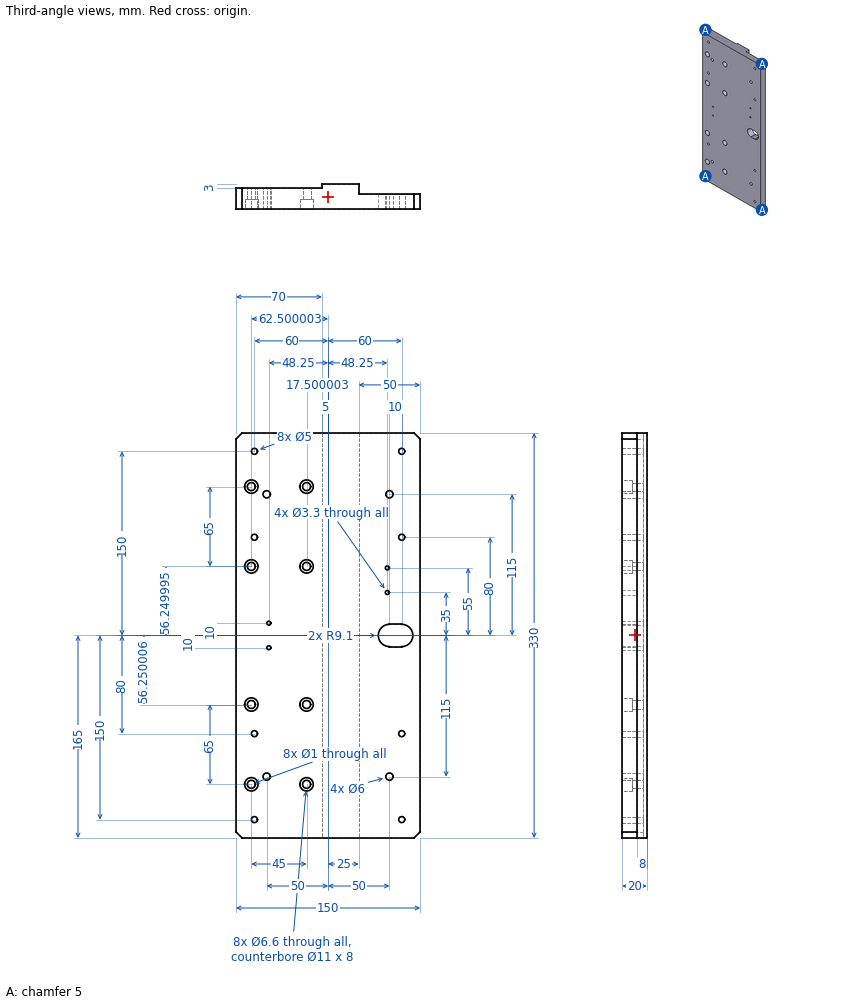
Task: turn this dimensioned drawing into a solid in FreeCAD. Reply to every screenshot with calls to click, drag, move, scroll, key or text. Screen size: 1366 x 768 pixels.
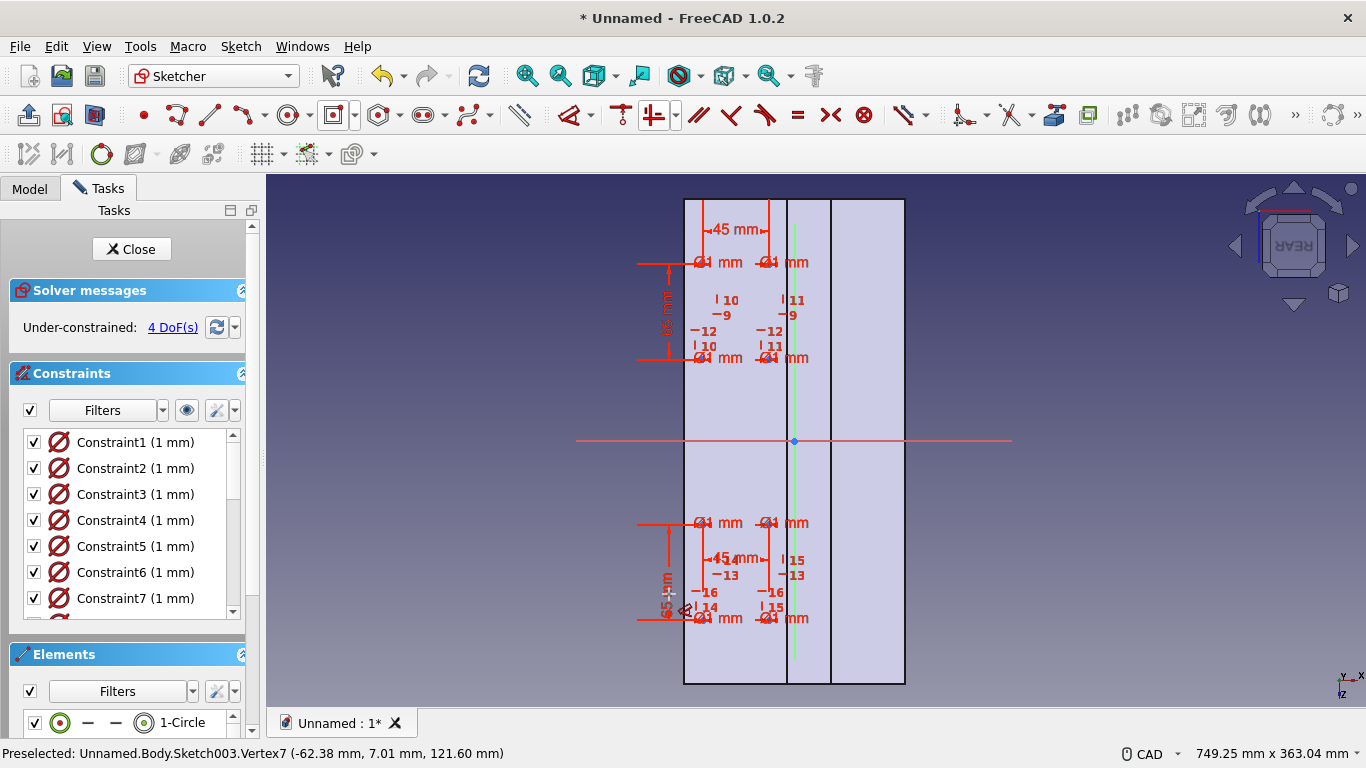
click(703, 264)
click(749, 475)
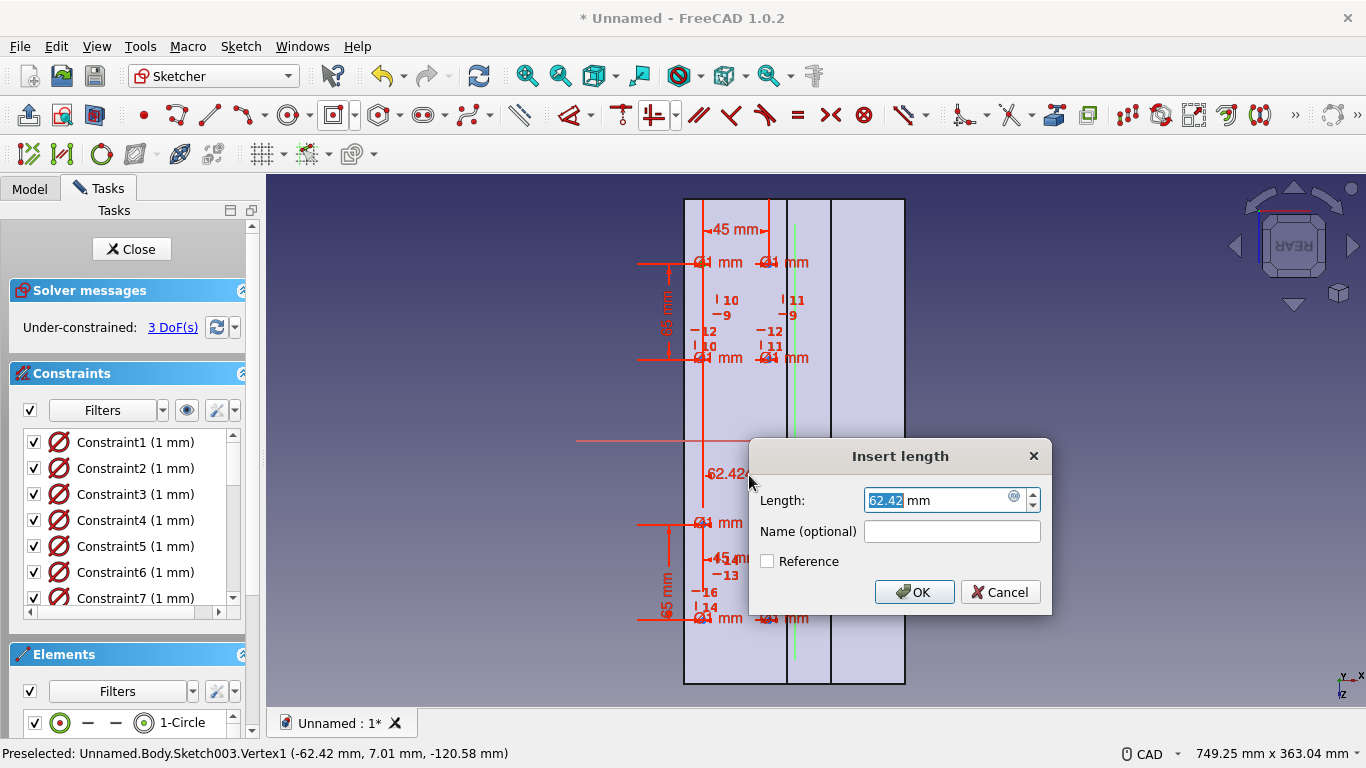
text(62.500006)
key(Return)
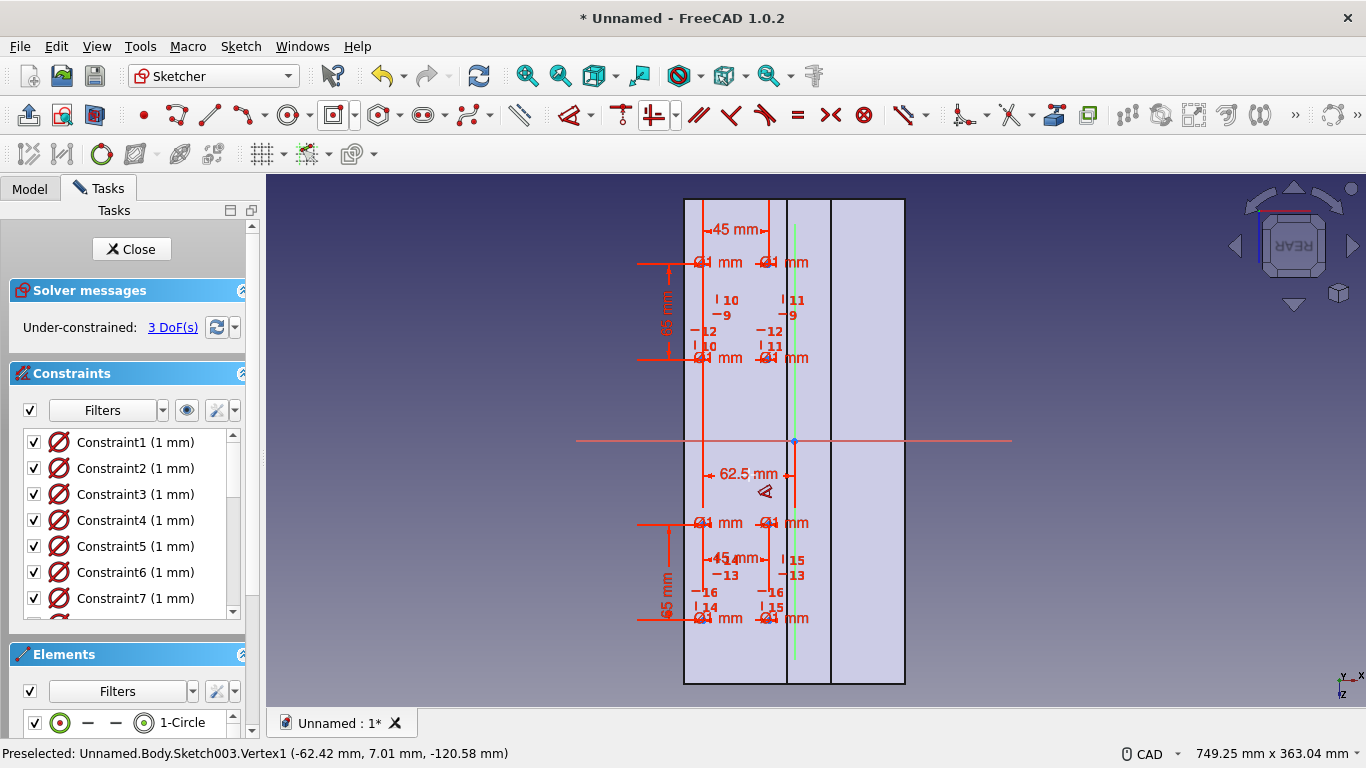
click(703, 360)
click(829, 401)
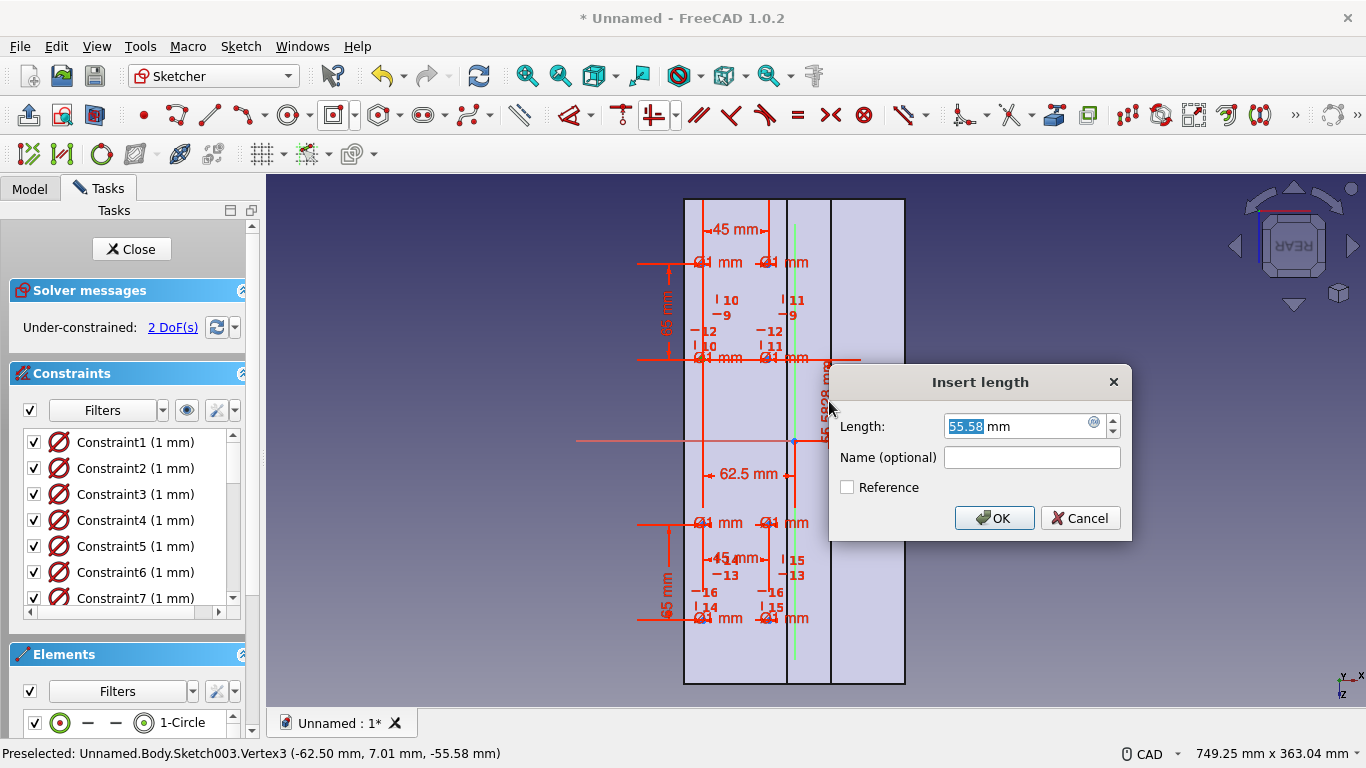
text(56.250006)
key(Return)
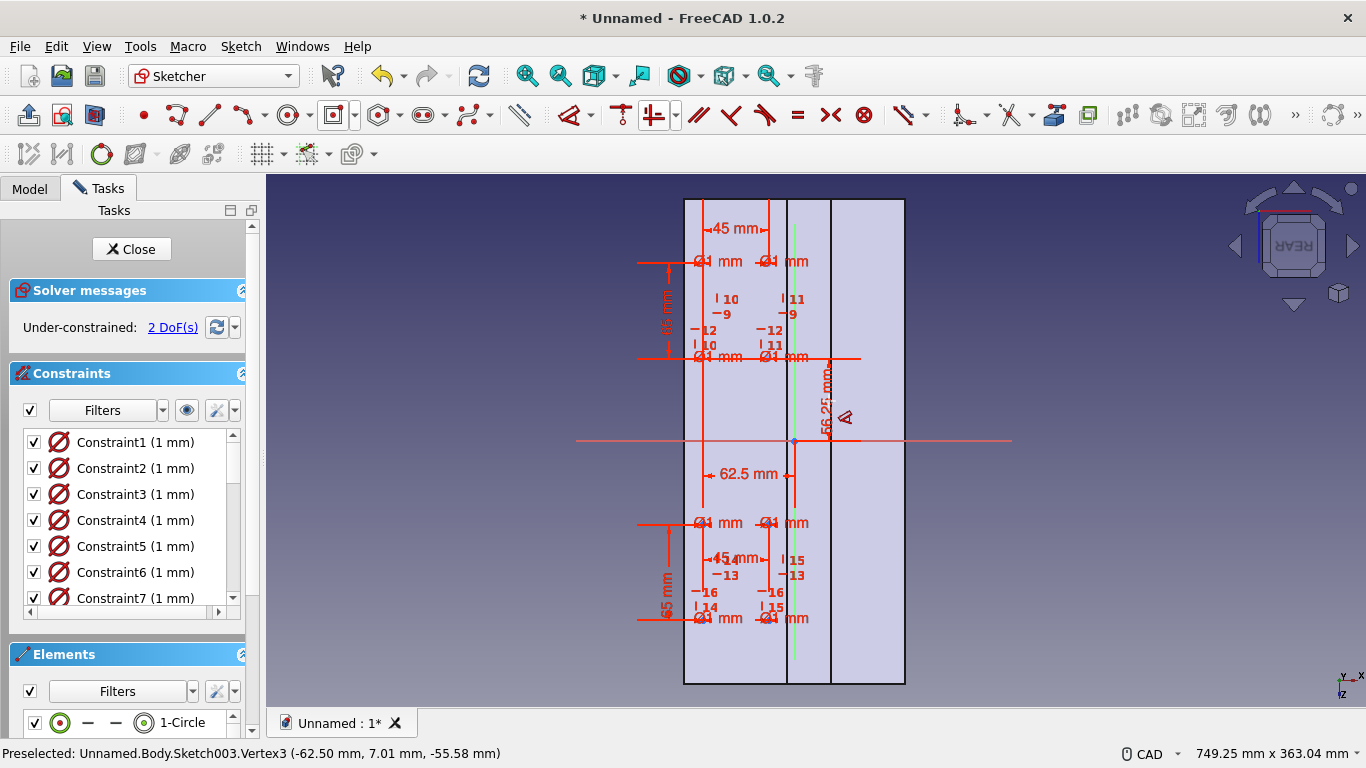
click(703, 525)
click(749, 407)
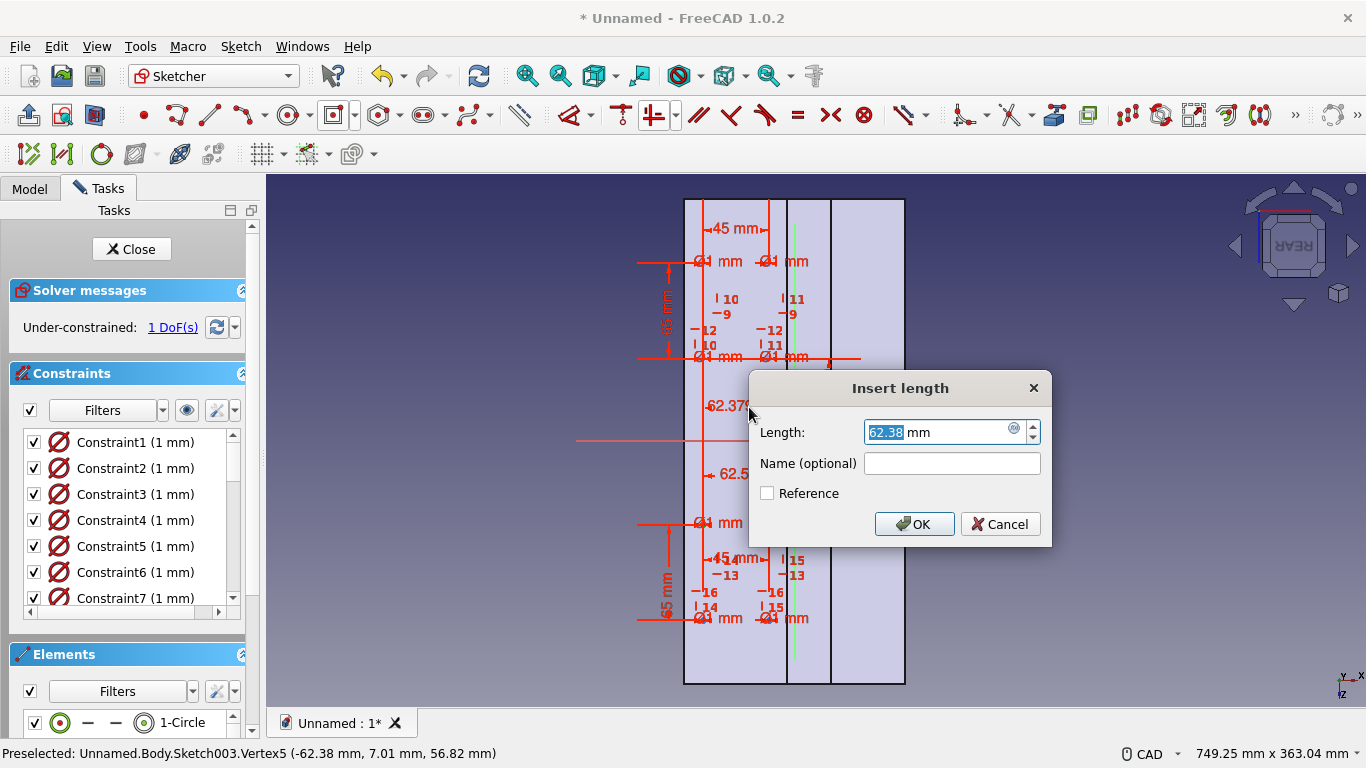
text(62.500003)
key(Return)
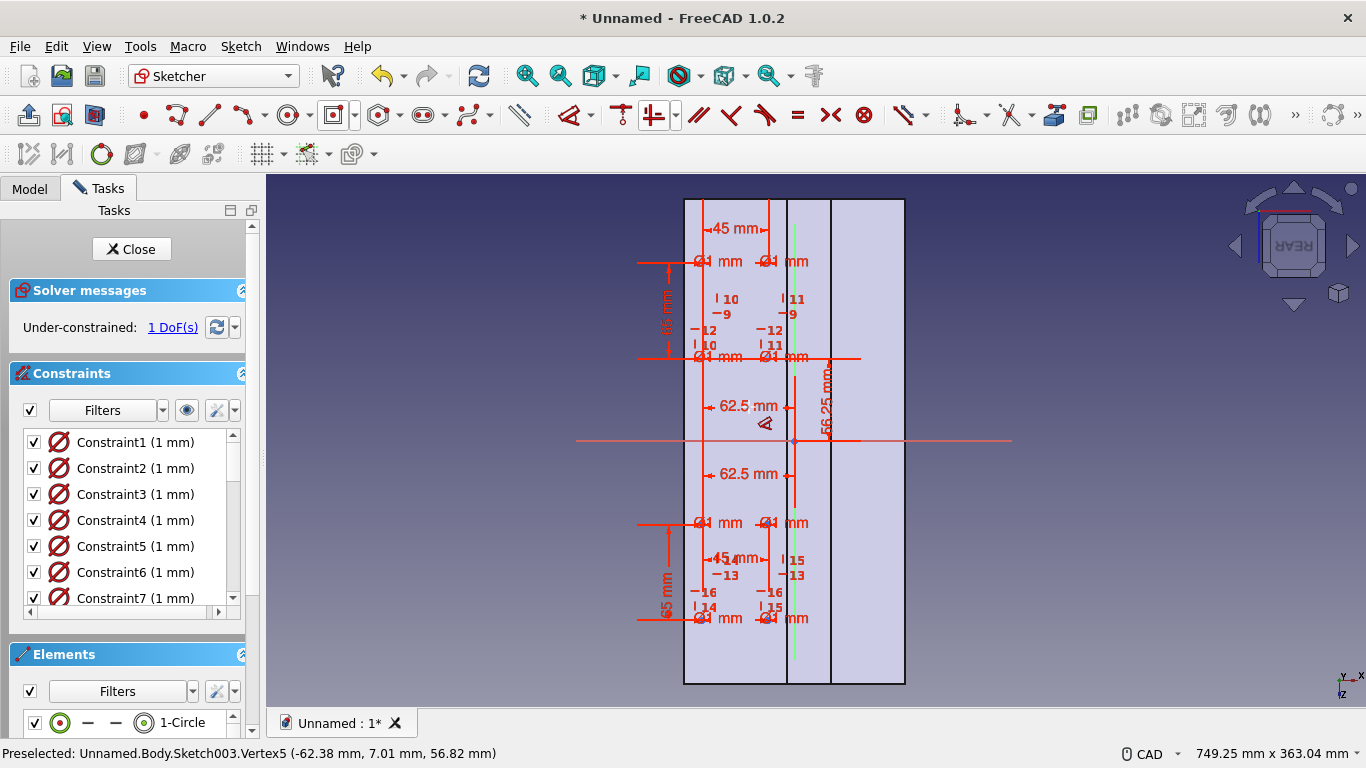
click(703, 525)
click(829, 483)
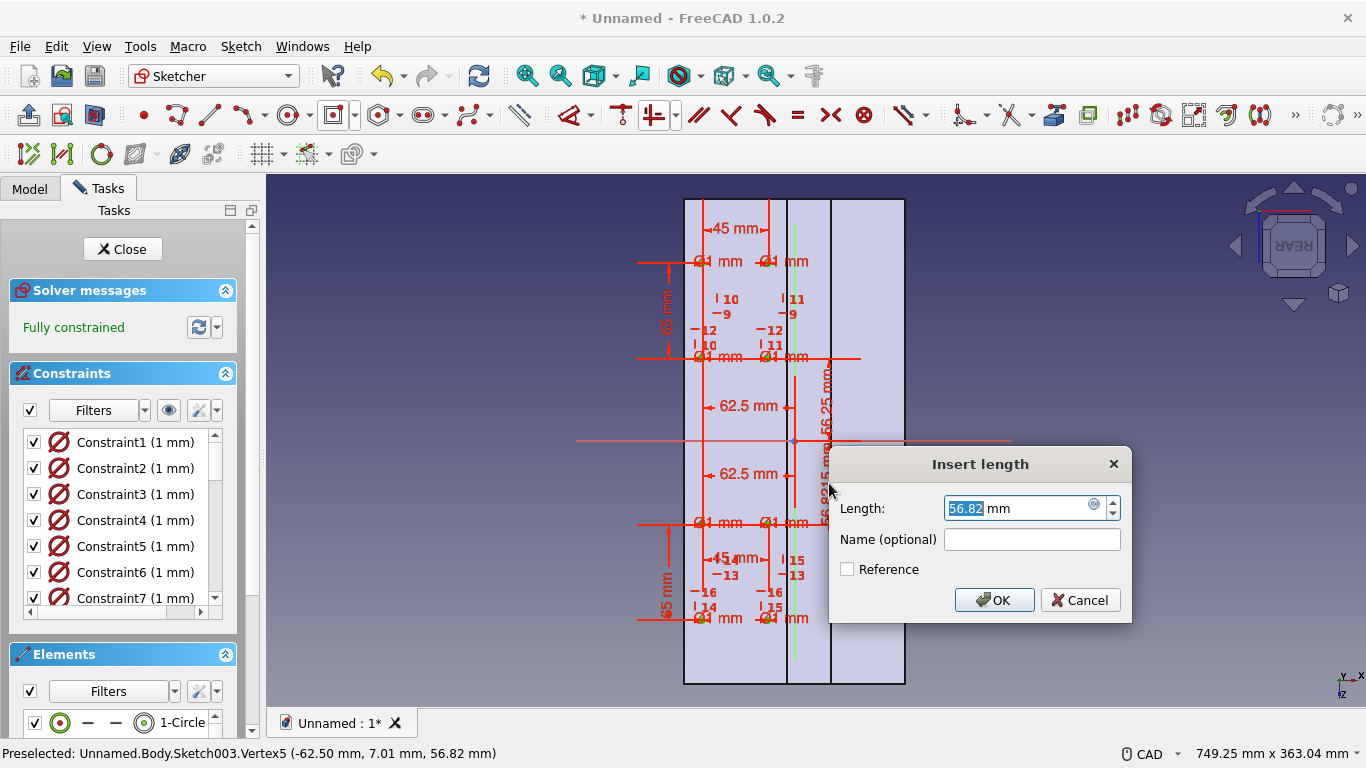
text(56.249995)
key(Return)
key(Escape)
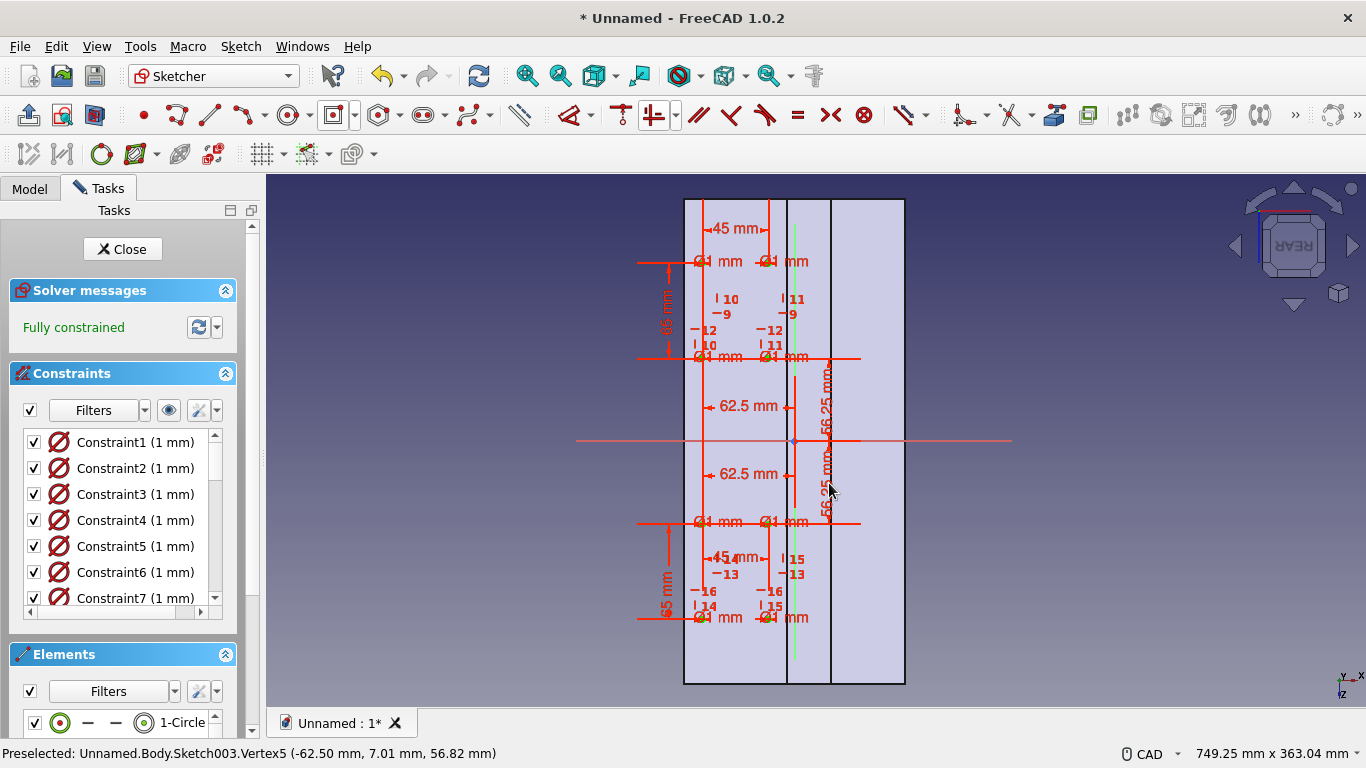
click(123, 249)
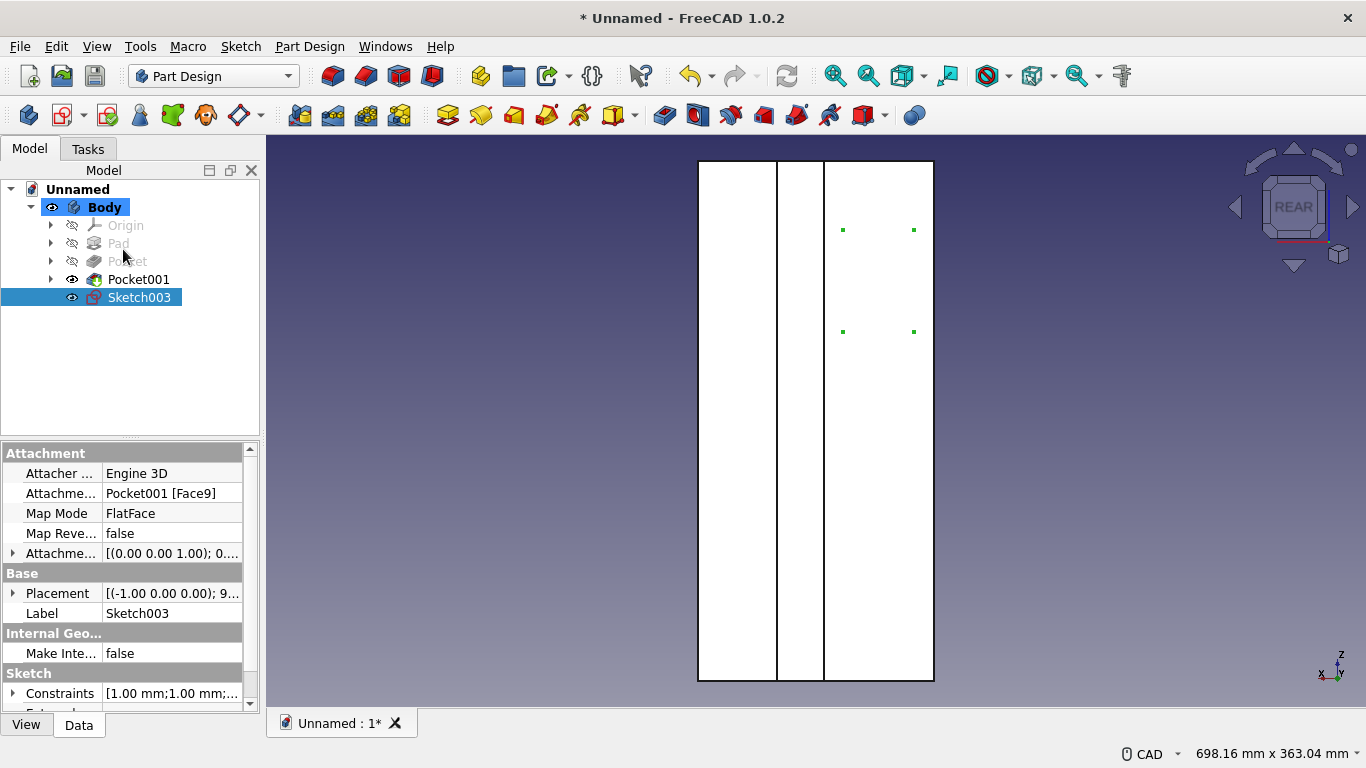
click(698, 116)